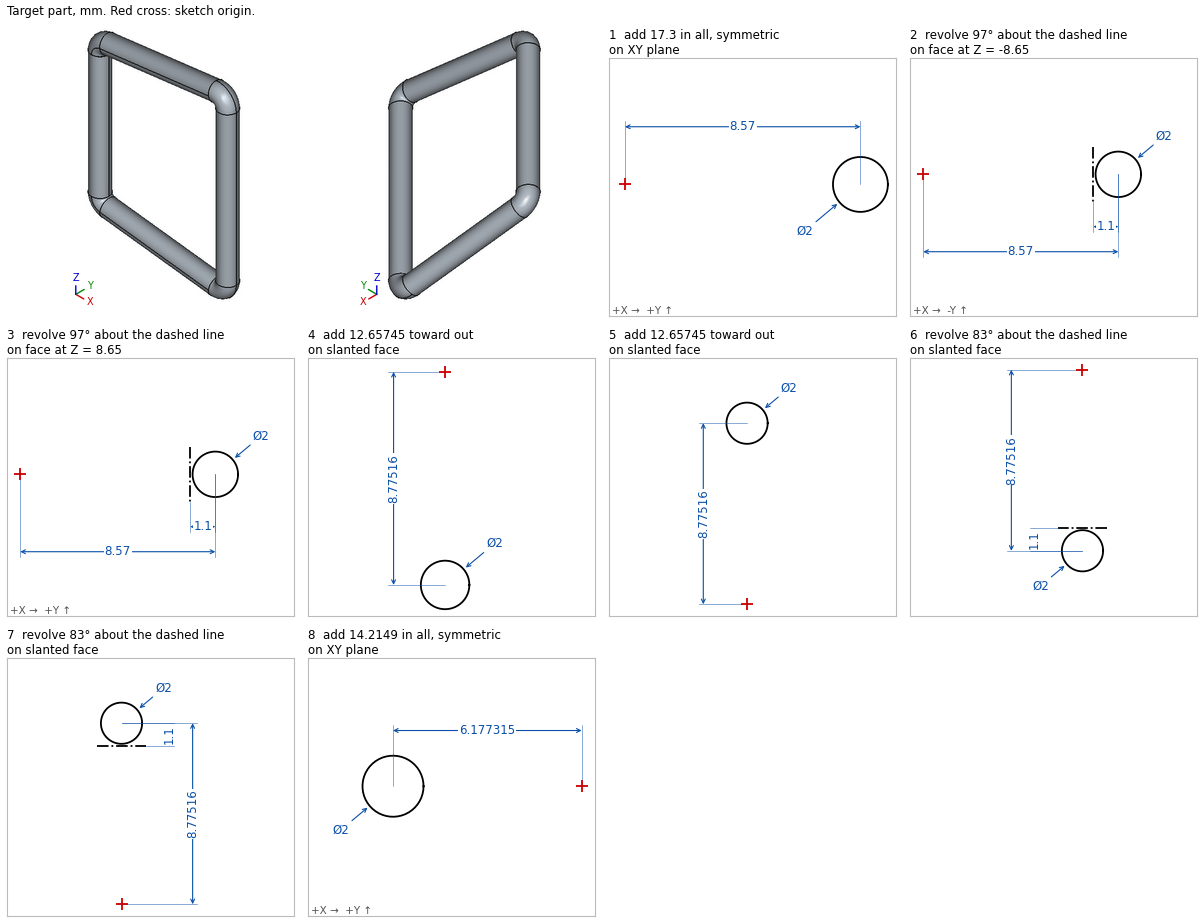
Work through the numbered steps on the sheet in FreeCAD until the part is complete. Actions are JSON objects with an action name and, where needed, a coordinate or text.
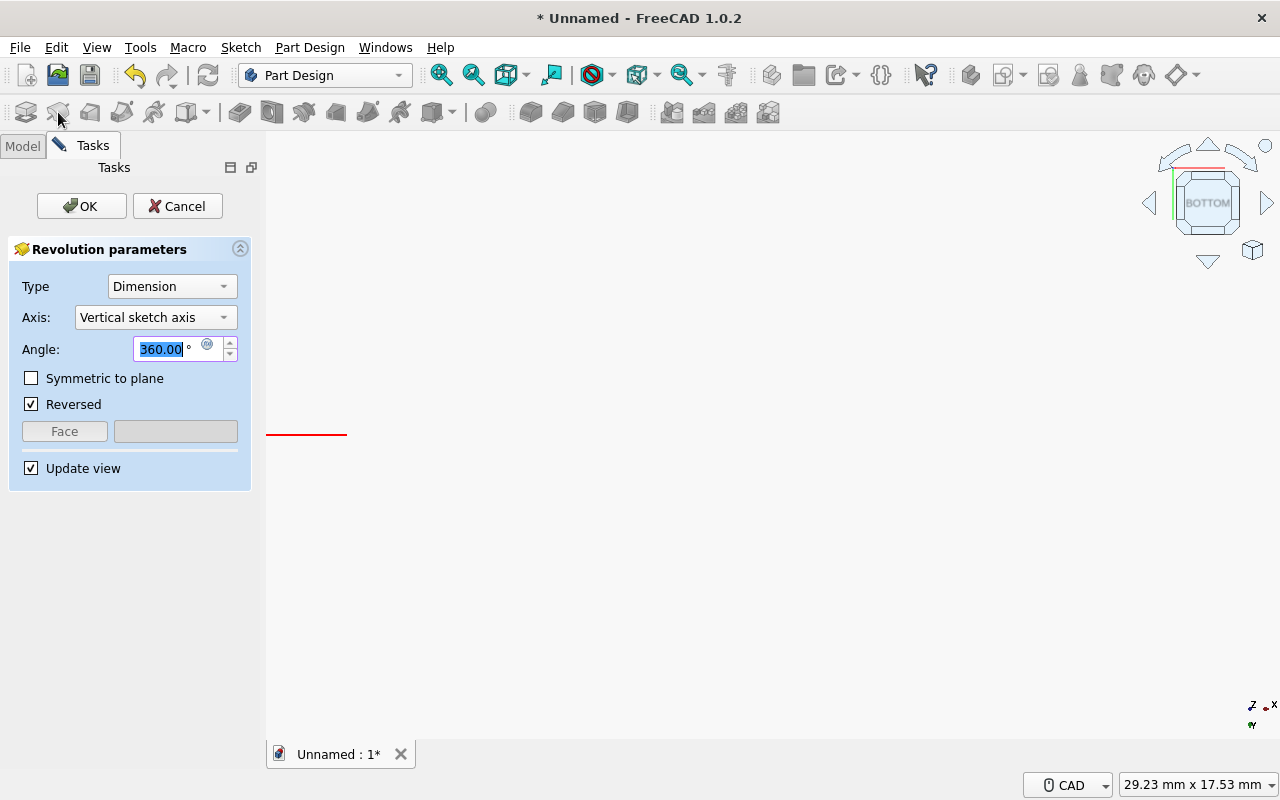
{"action": "left_click", "coordinate": [156, 318]}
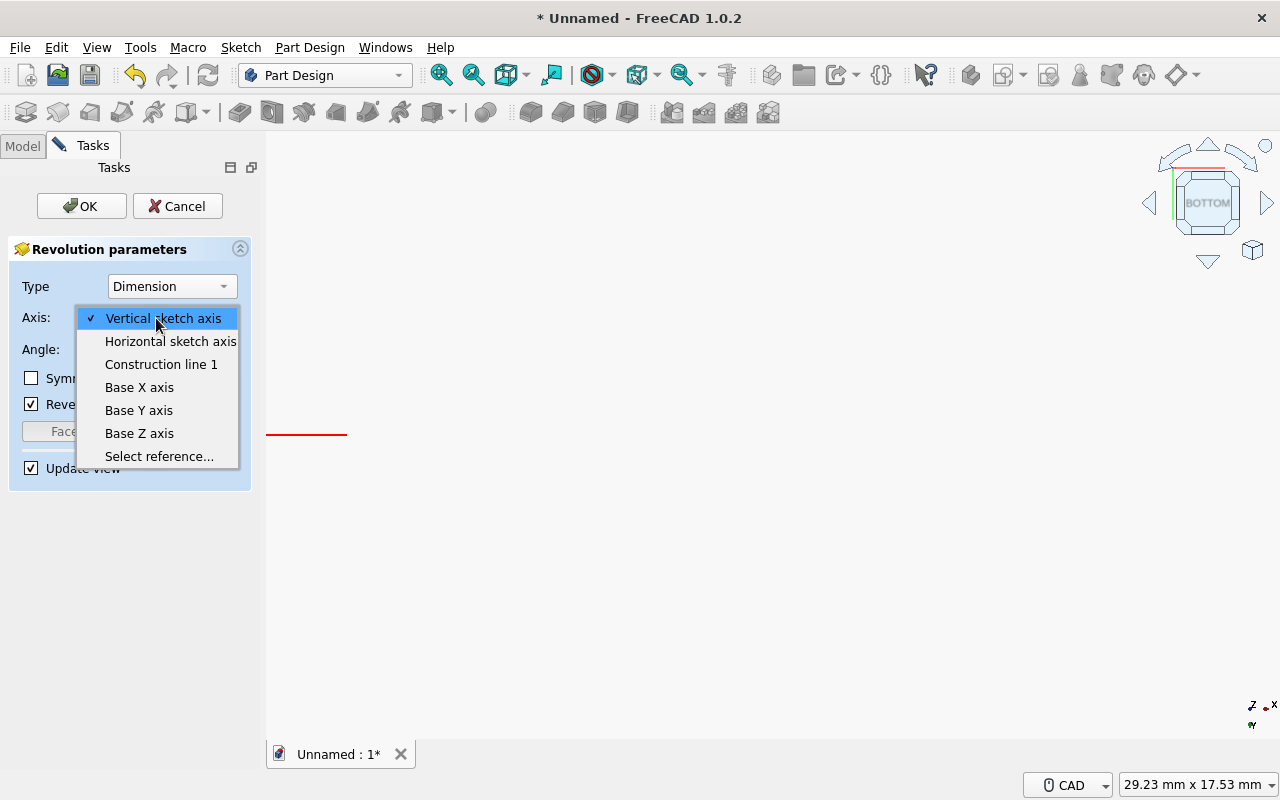
{"action": "left_click", "coordinate": [156, 364]}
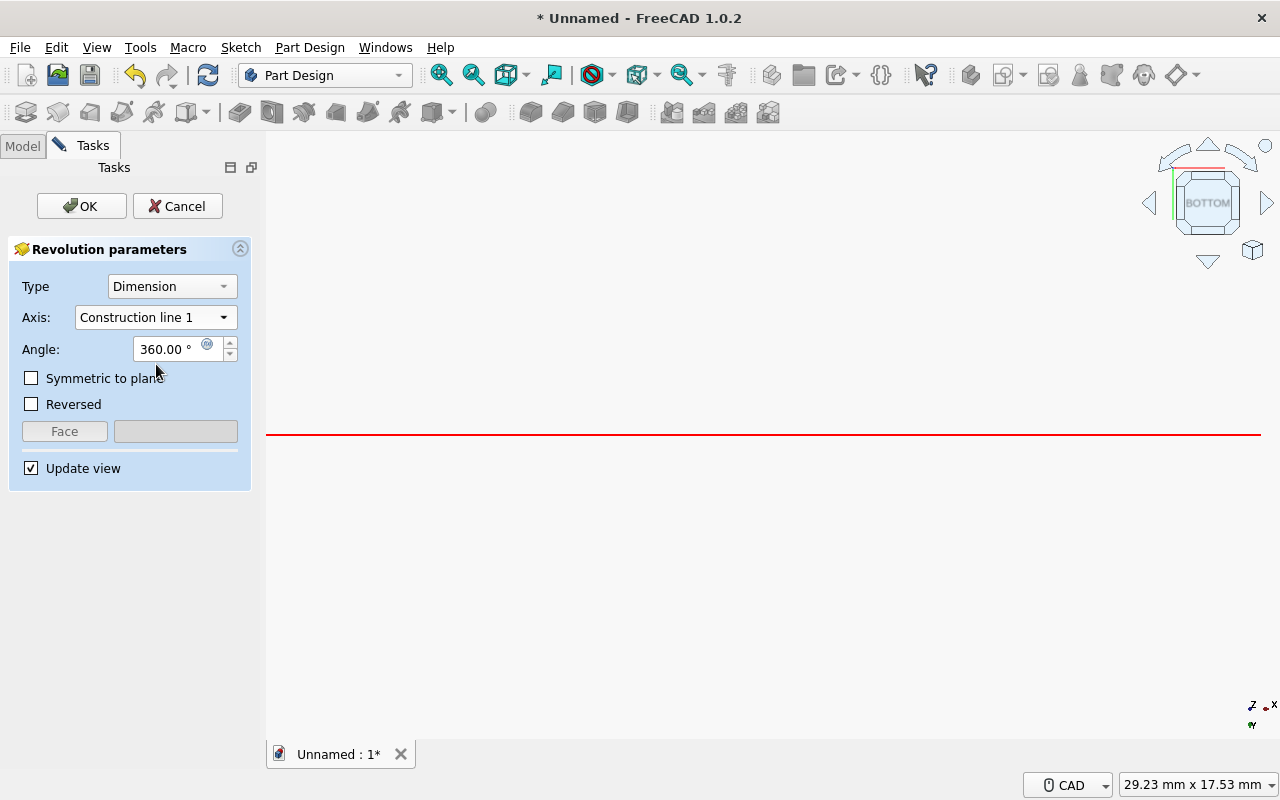
{"action": "triple_click", "coordinate": [178, 349]}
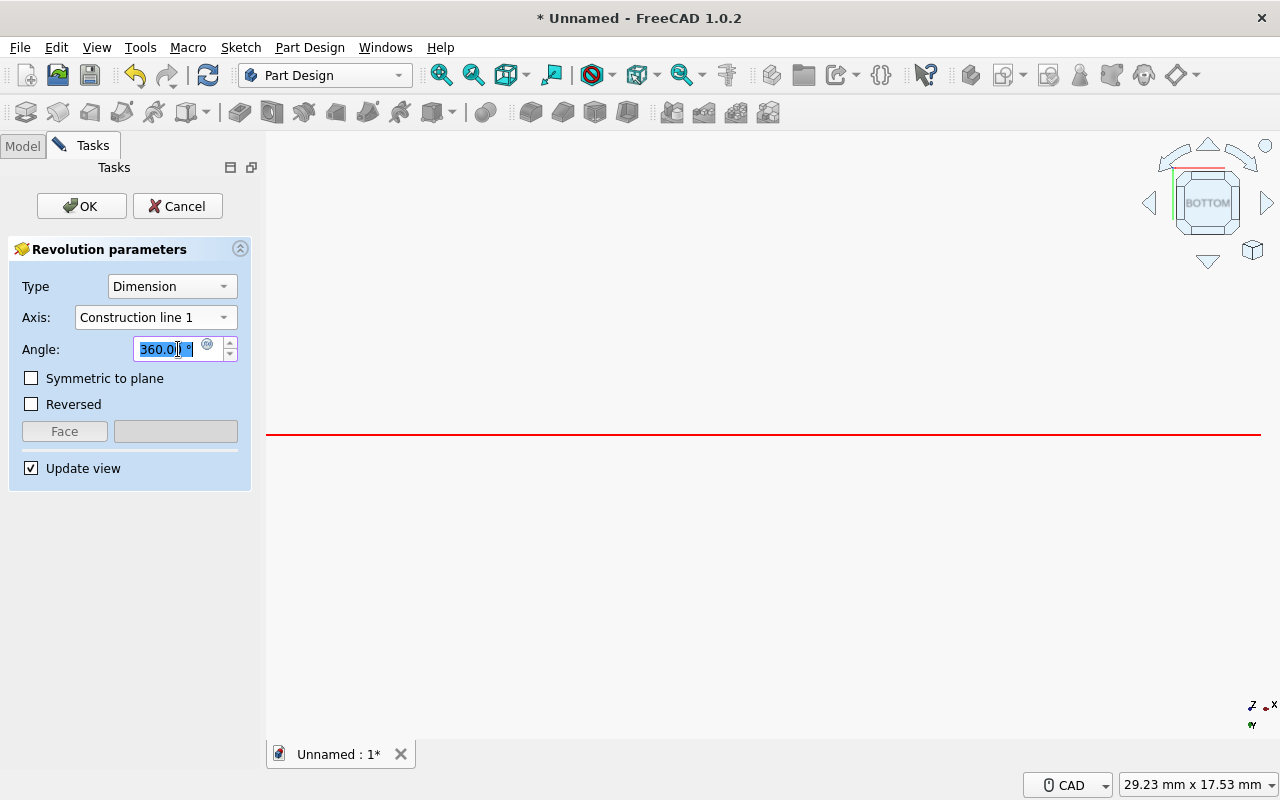
{"action": "type", "text": "97"}
{"action": "key", "text": "Tab"}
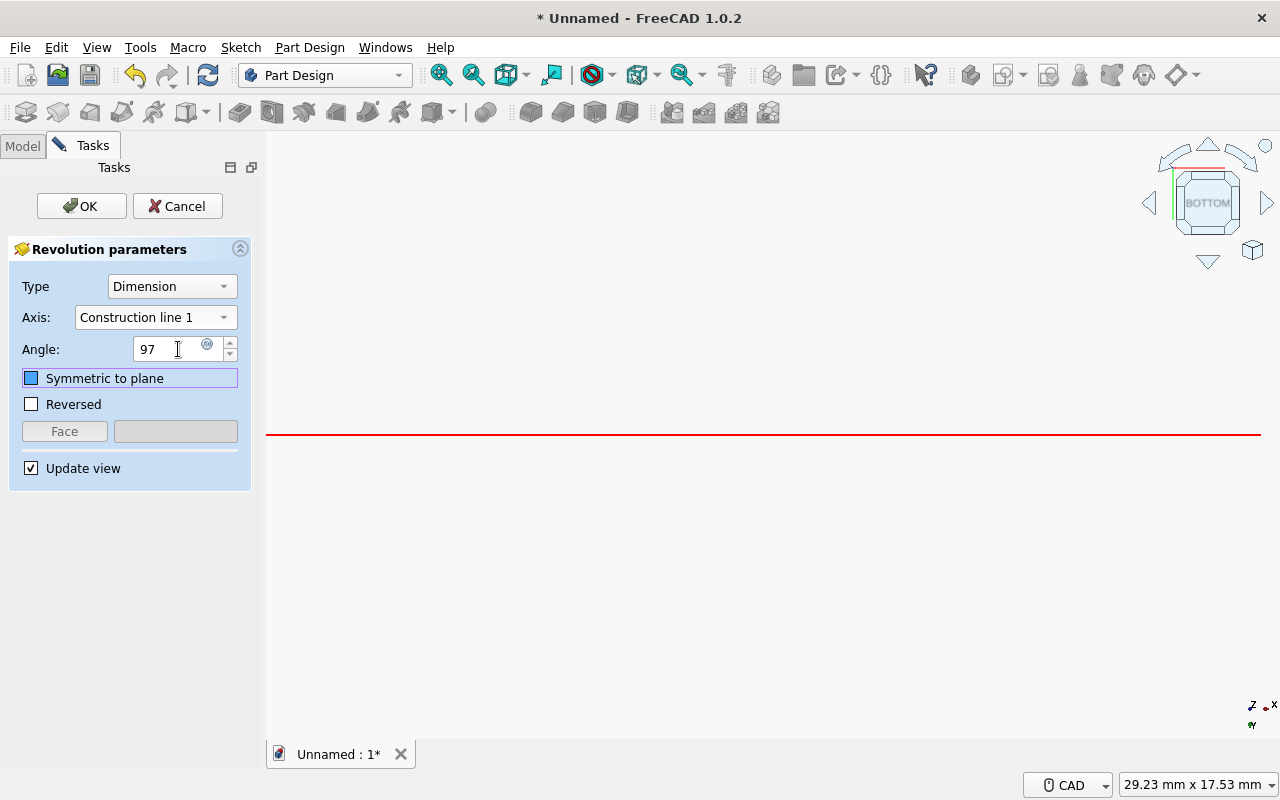
{"action": "left_click", "coordinate": [82, 206]}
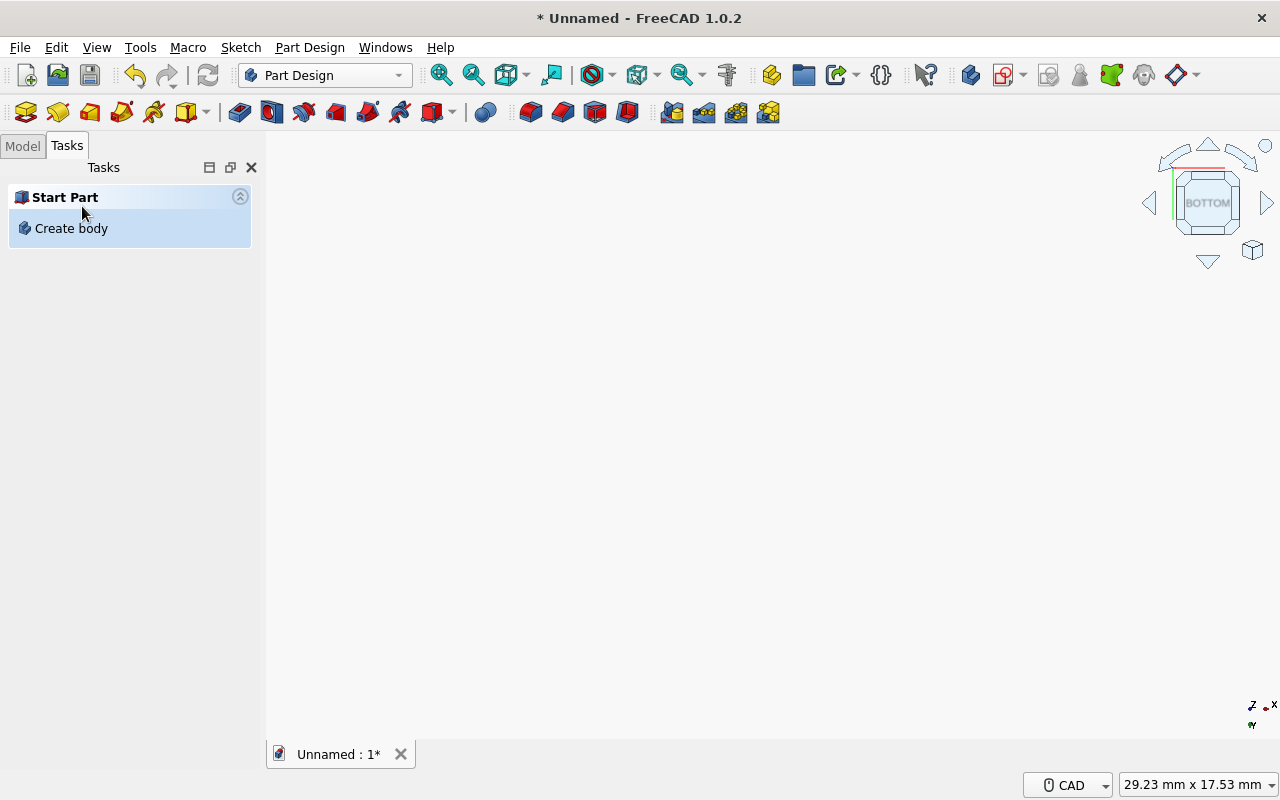
{"action": "left_click", "coordinate": [442, 76]}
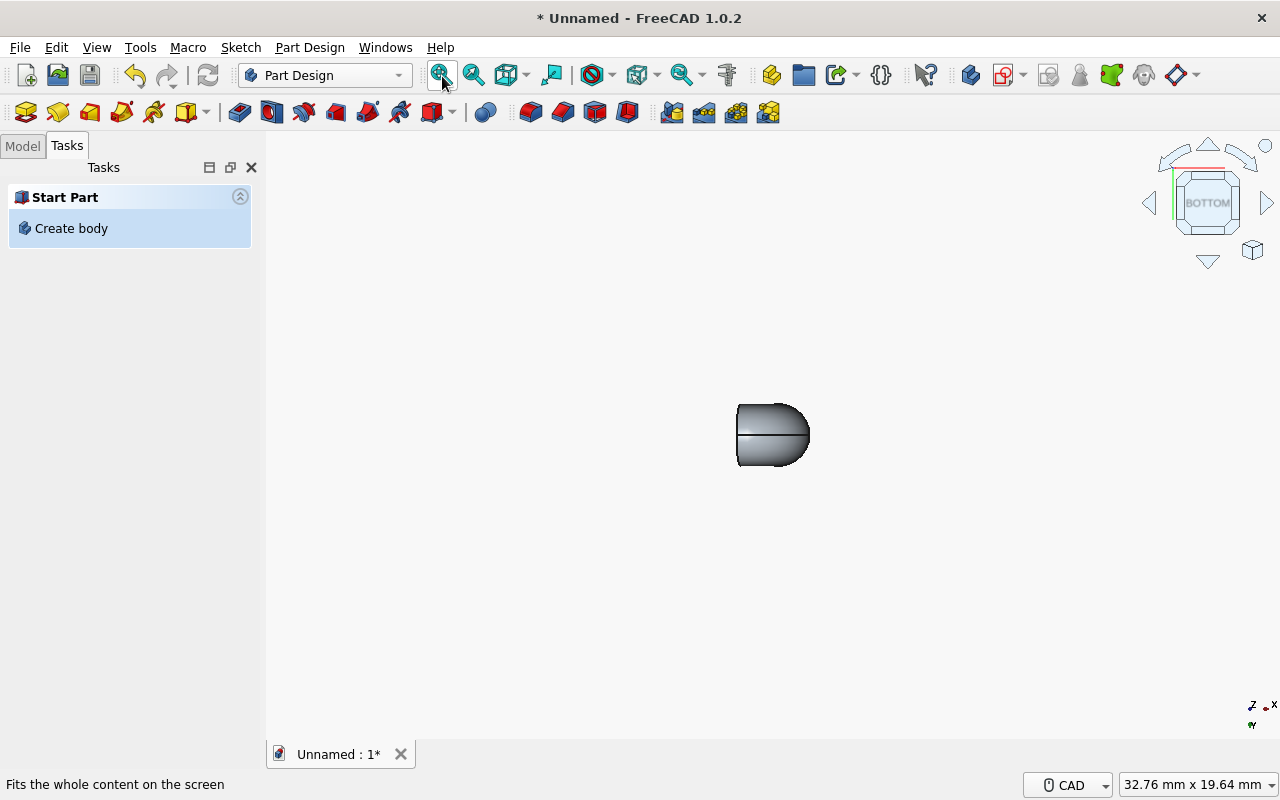
{"action": "key", "text": "0"}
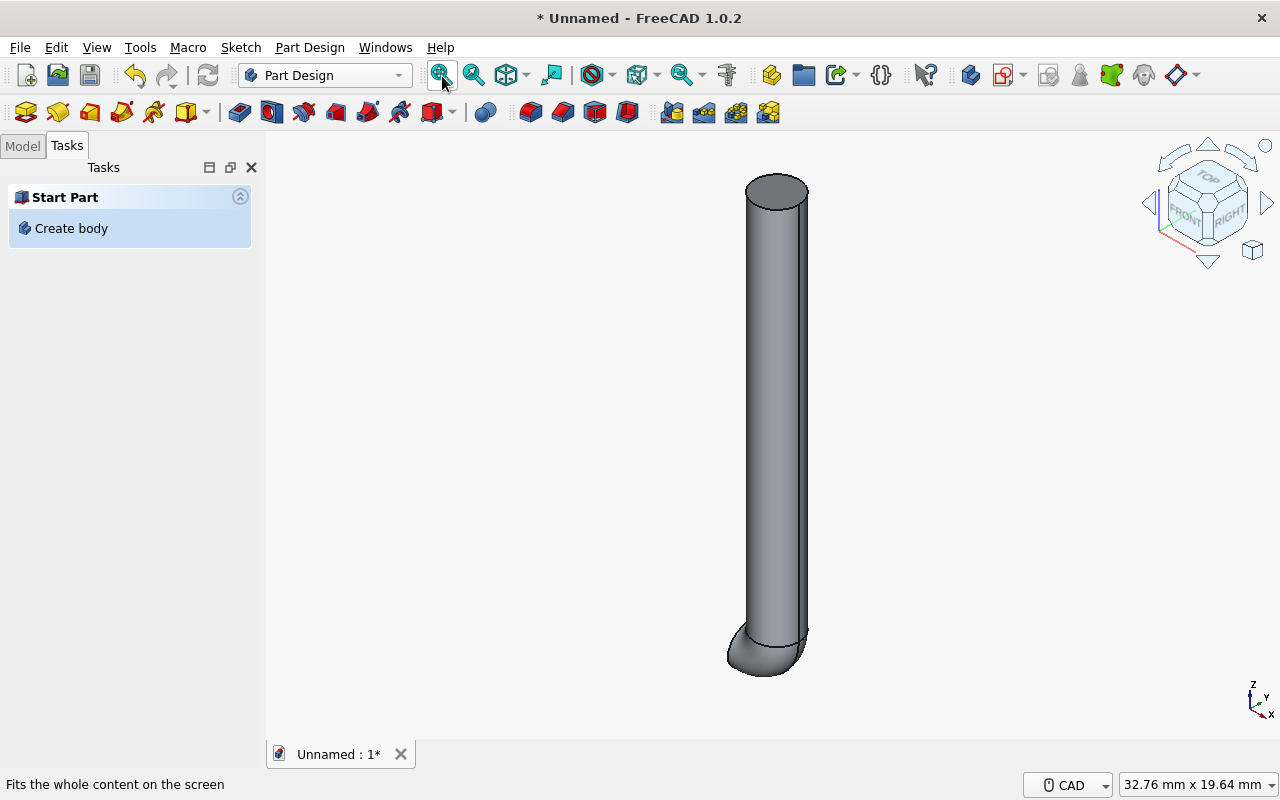
{"action": "left_click", "coordinate": [777, 191]}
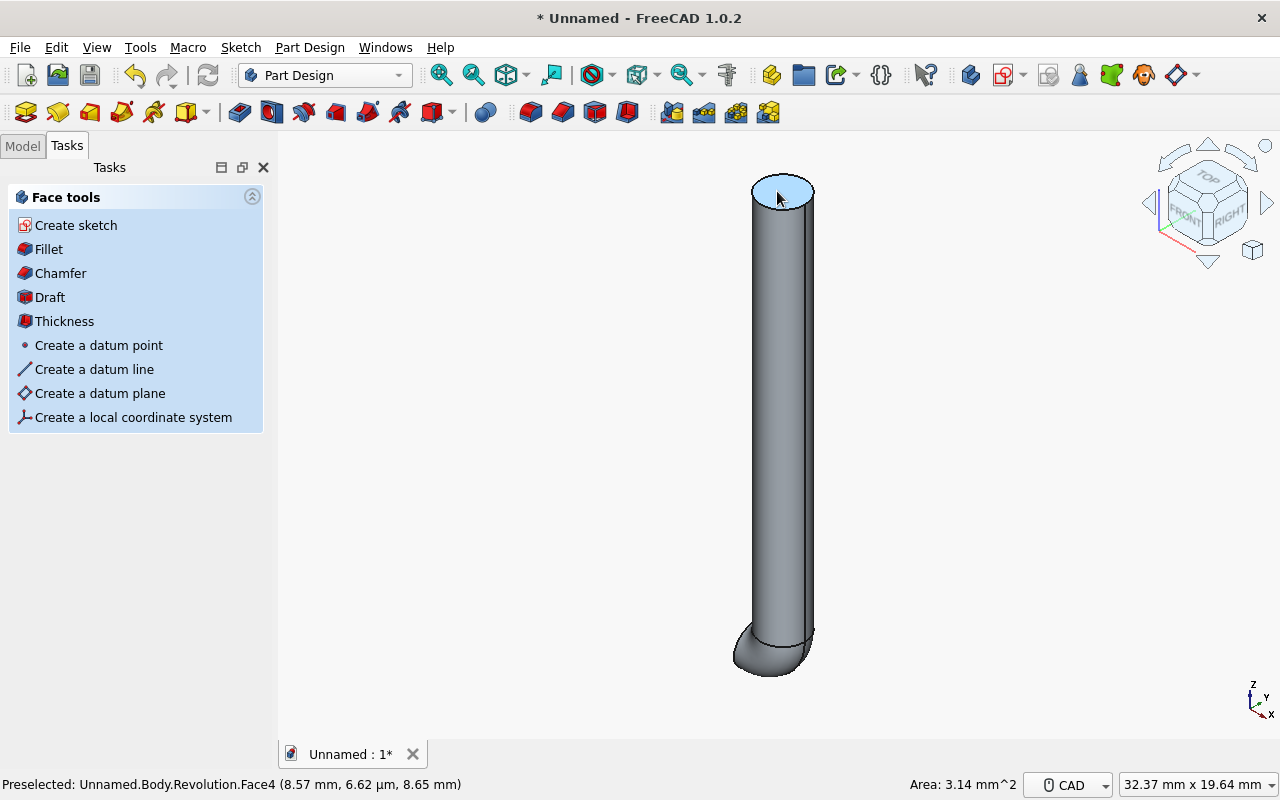
{"action": "left_click", "coordinate": [1004, 76]}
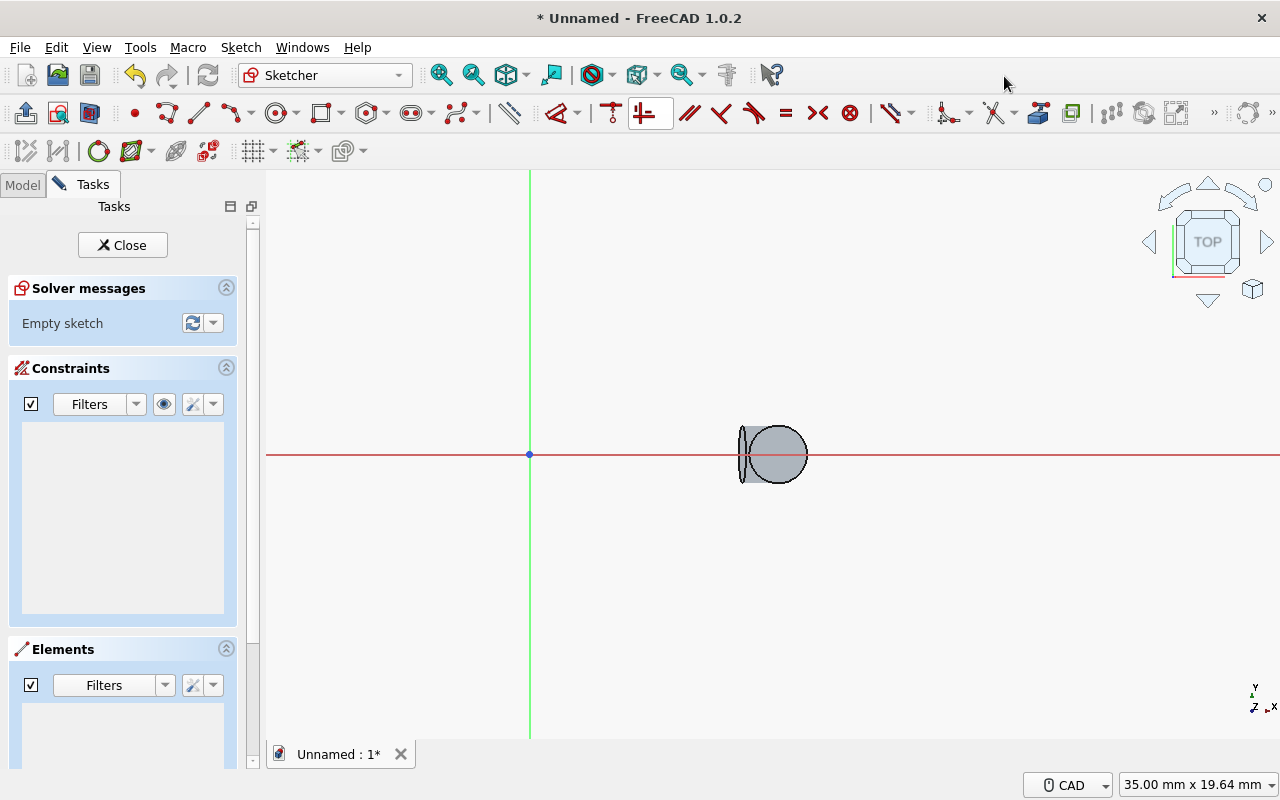
{"action": "scroll", "coordinate": [795, 455], "scroll_direction": "up", "scroll_amount": 8}